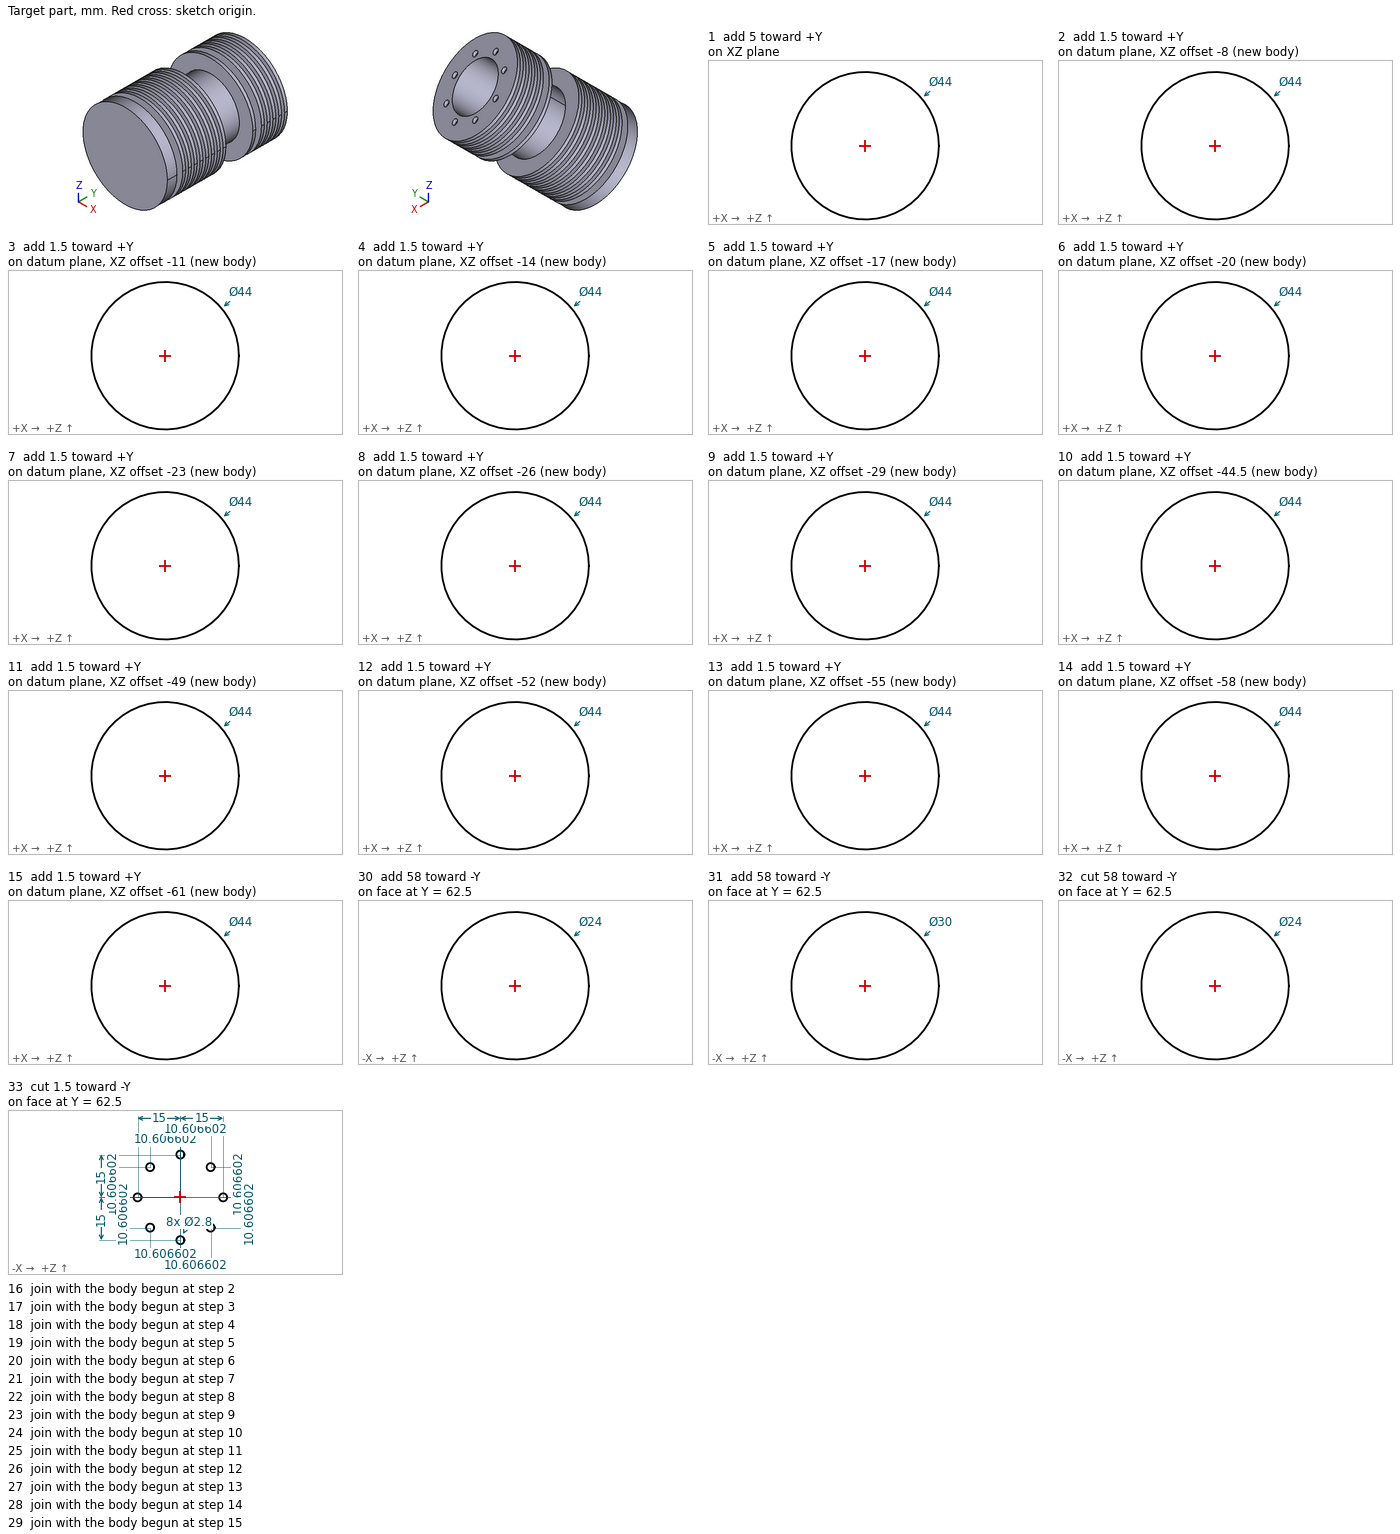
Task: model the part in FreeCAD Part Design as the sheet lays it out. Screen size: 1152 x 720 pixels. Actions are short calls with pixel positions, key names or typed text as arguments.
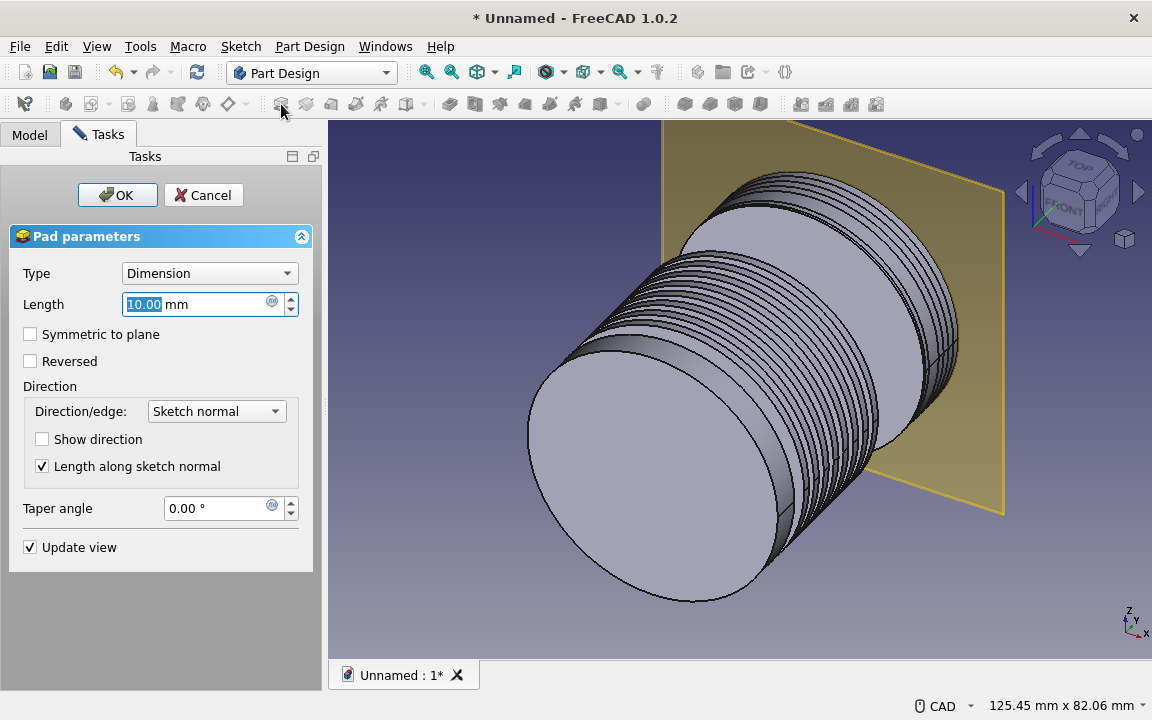
text(1.5)
key(Tab)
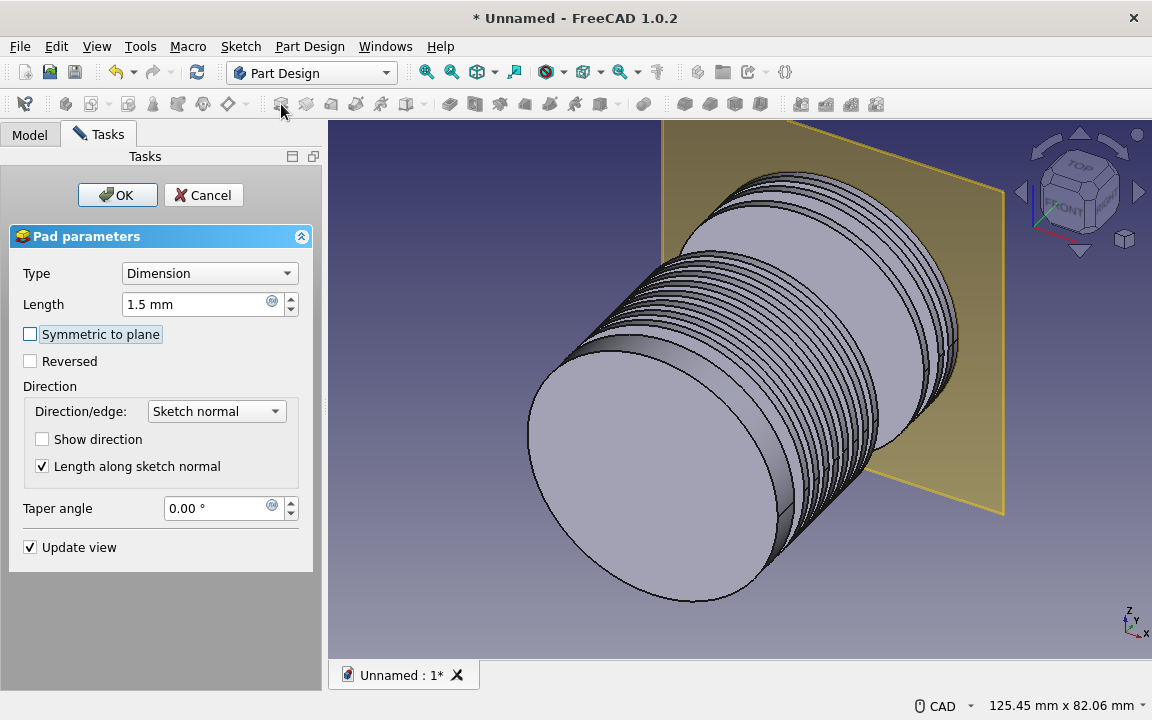
click(31, 361)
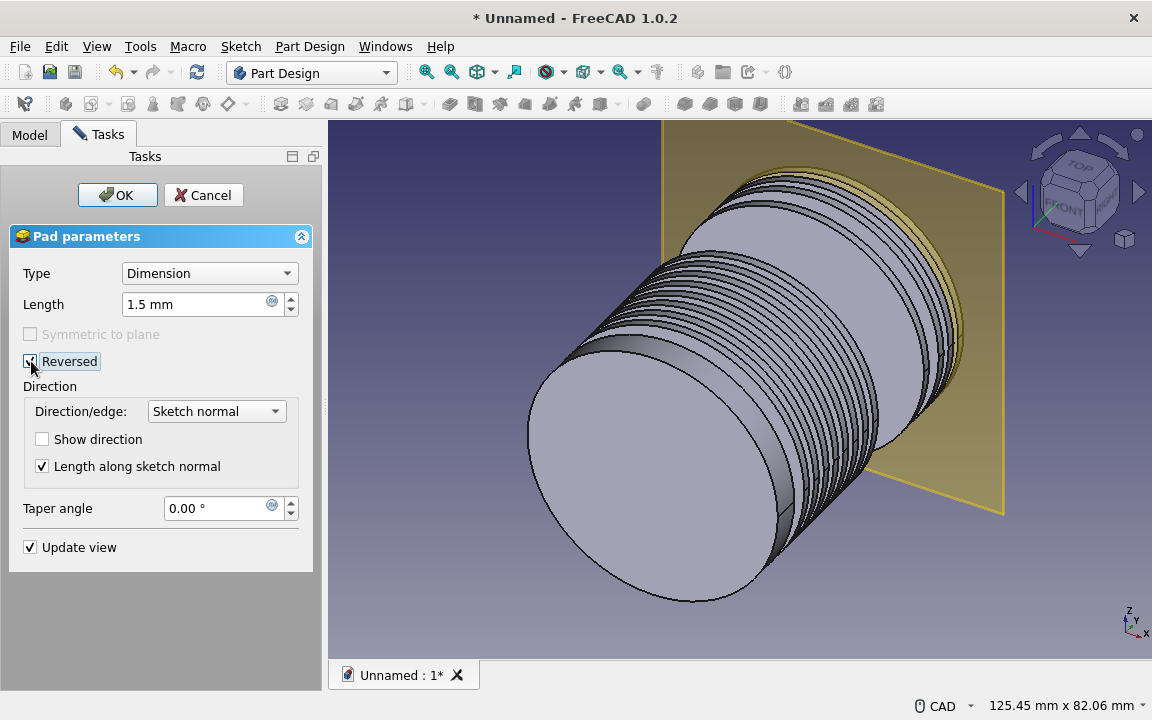
click(118, 195)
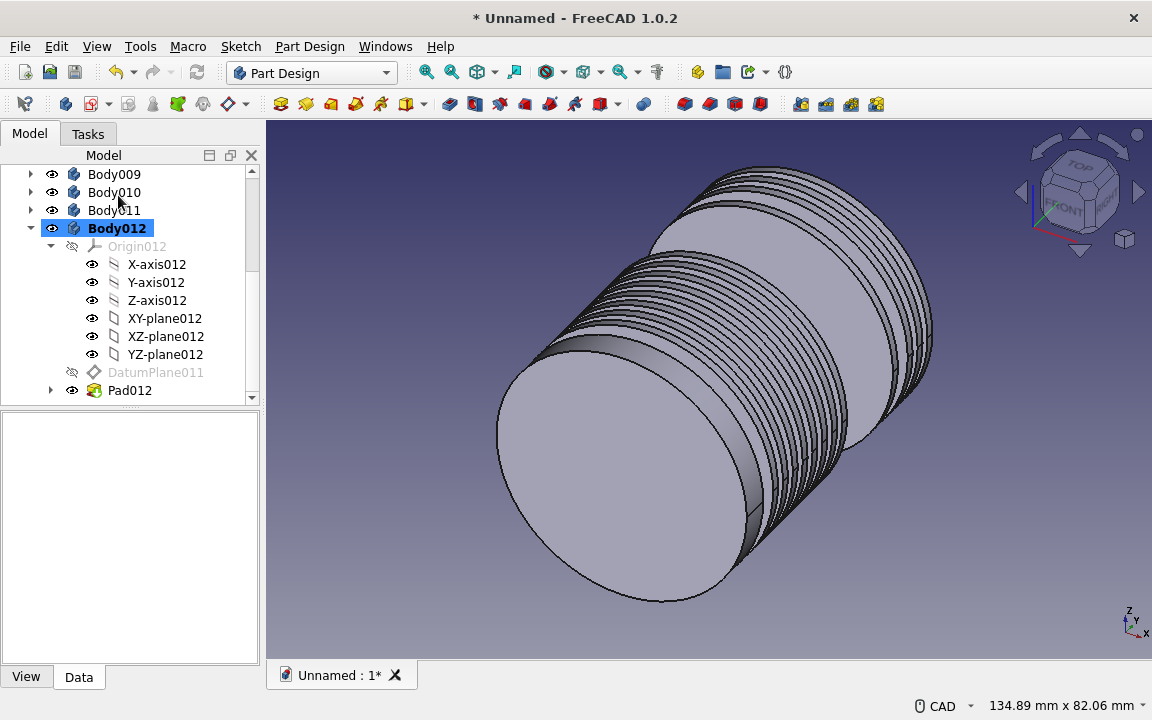
click(66, 104)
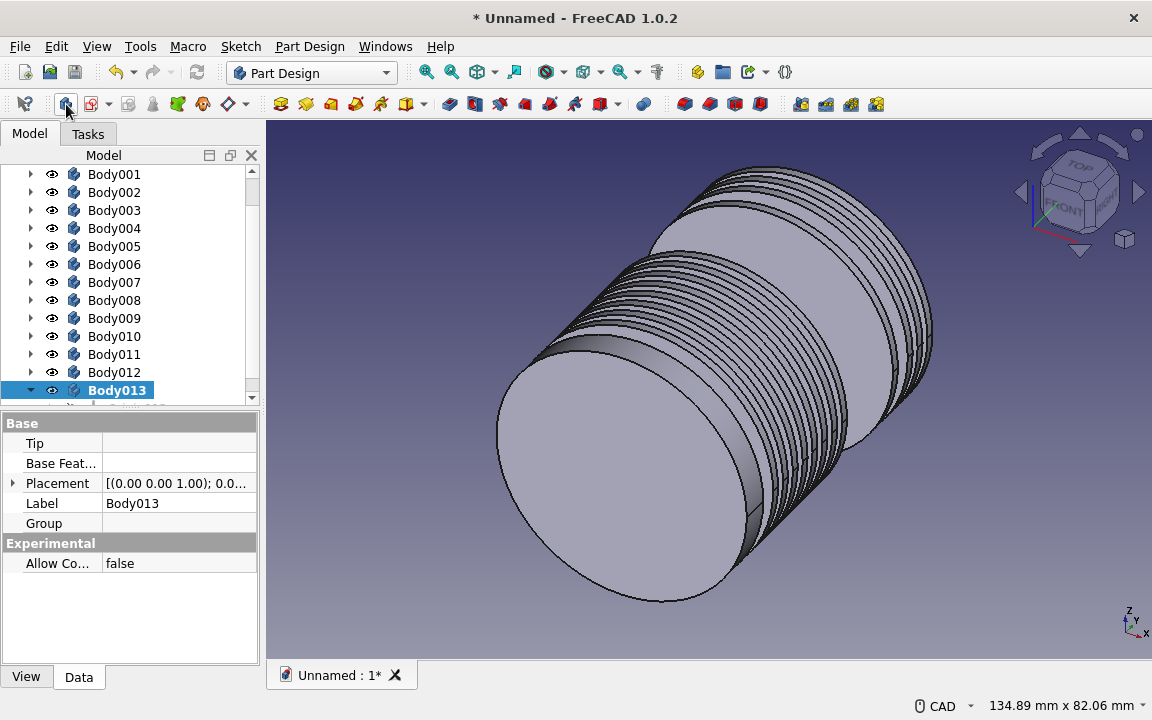
scroll(121, 278, down, 3)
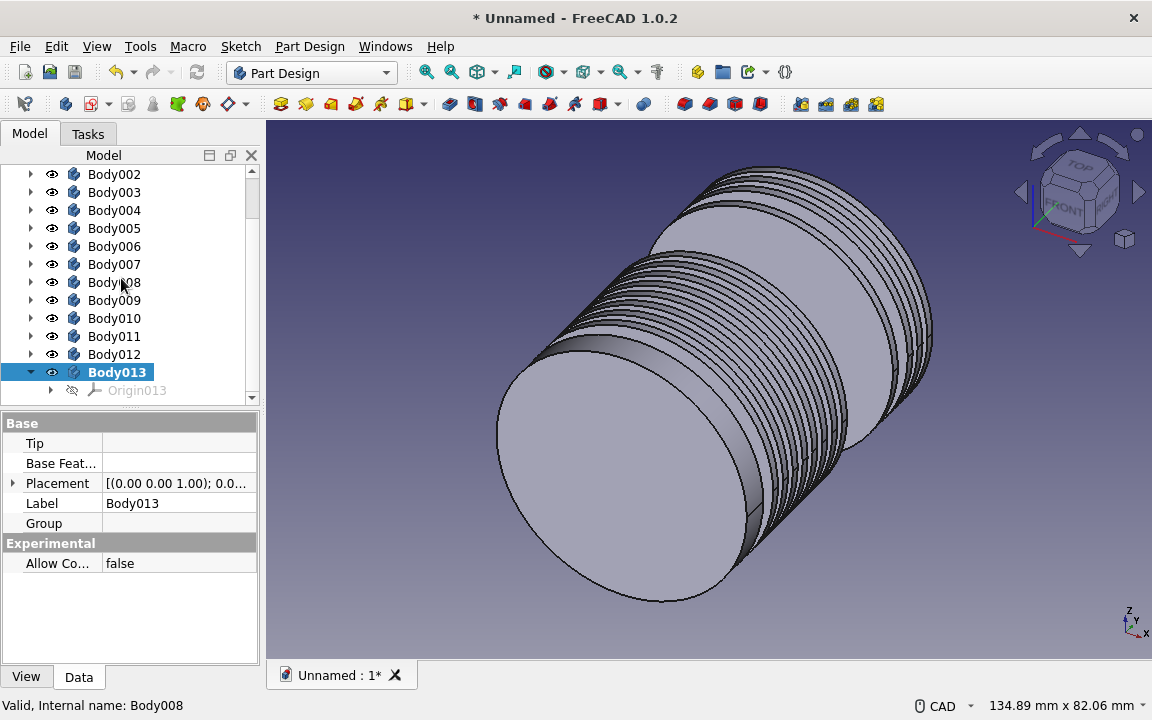
click(51, 390)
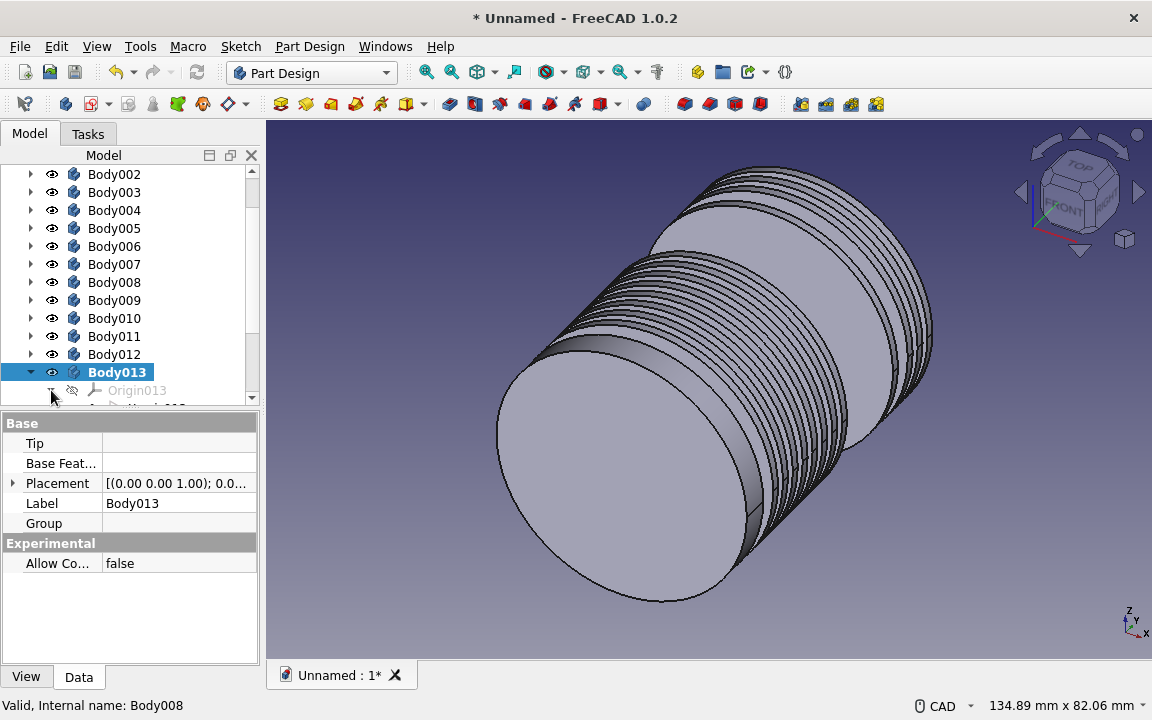
scroll(121, 278, down, 3)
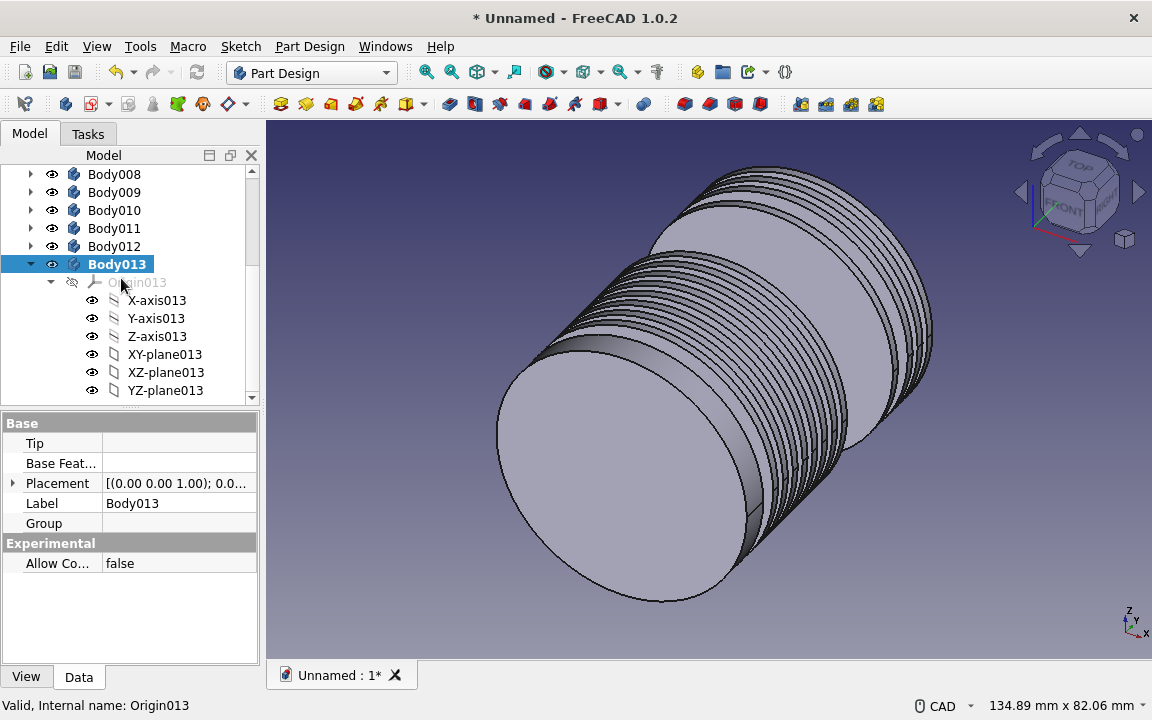
click(137, 372)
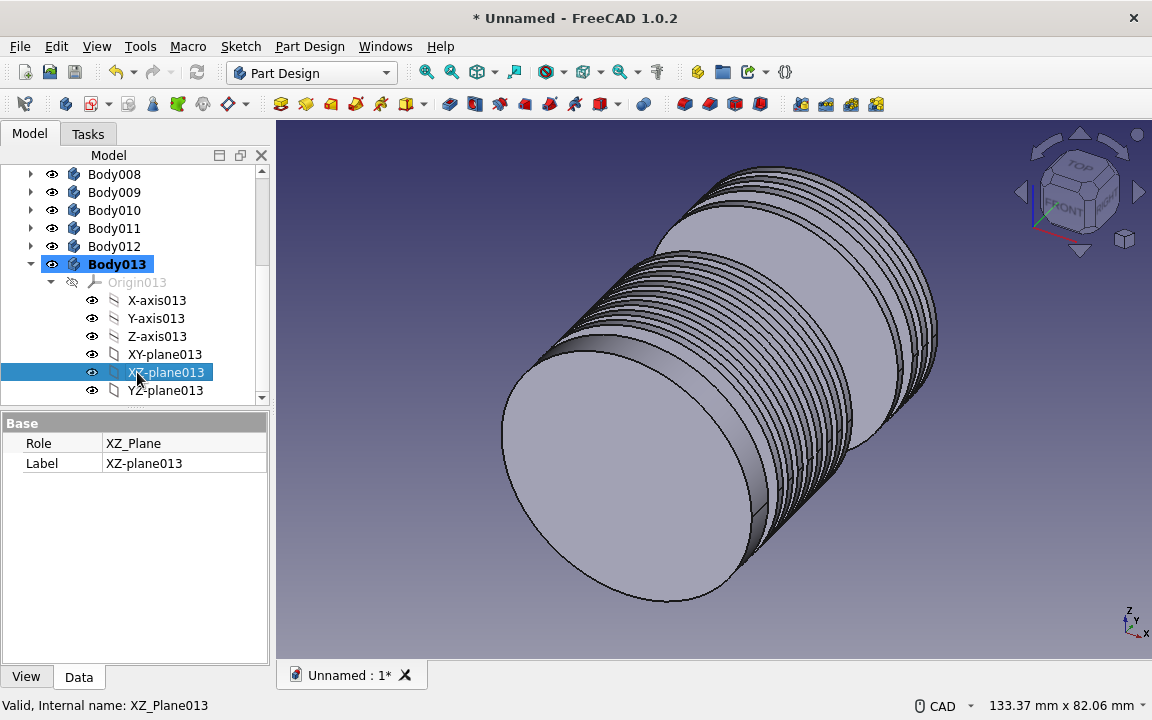
click(228, 104)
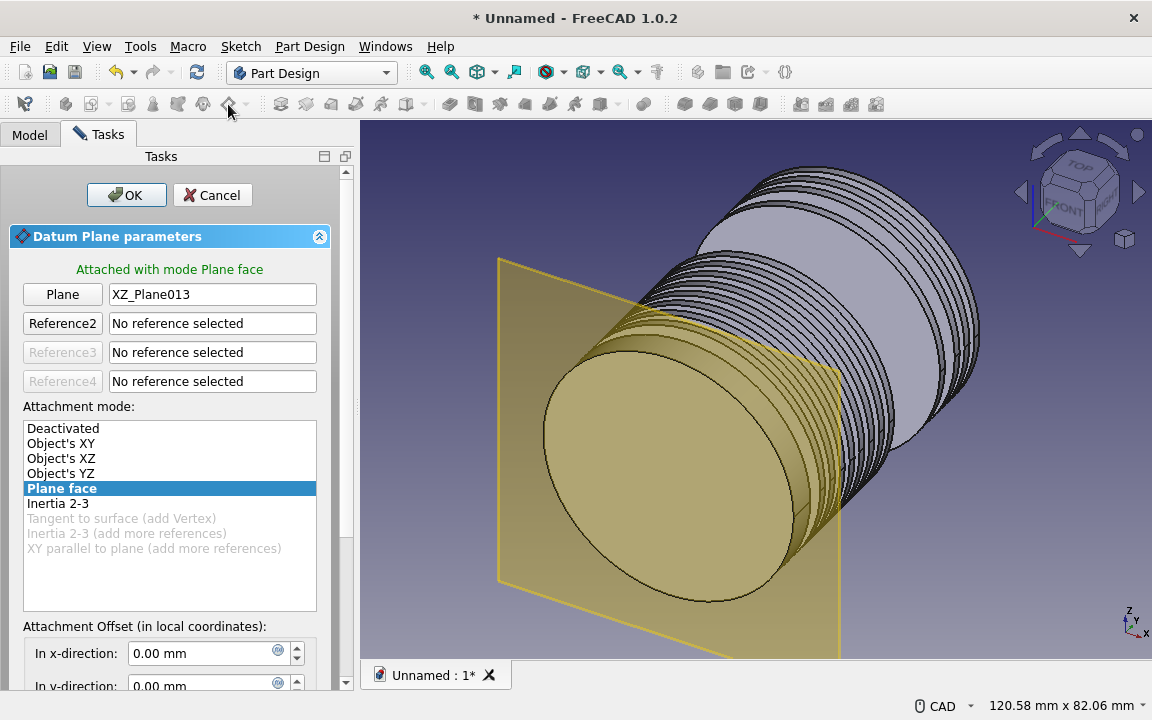
scroll(346, 428, down, 2)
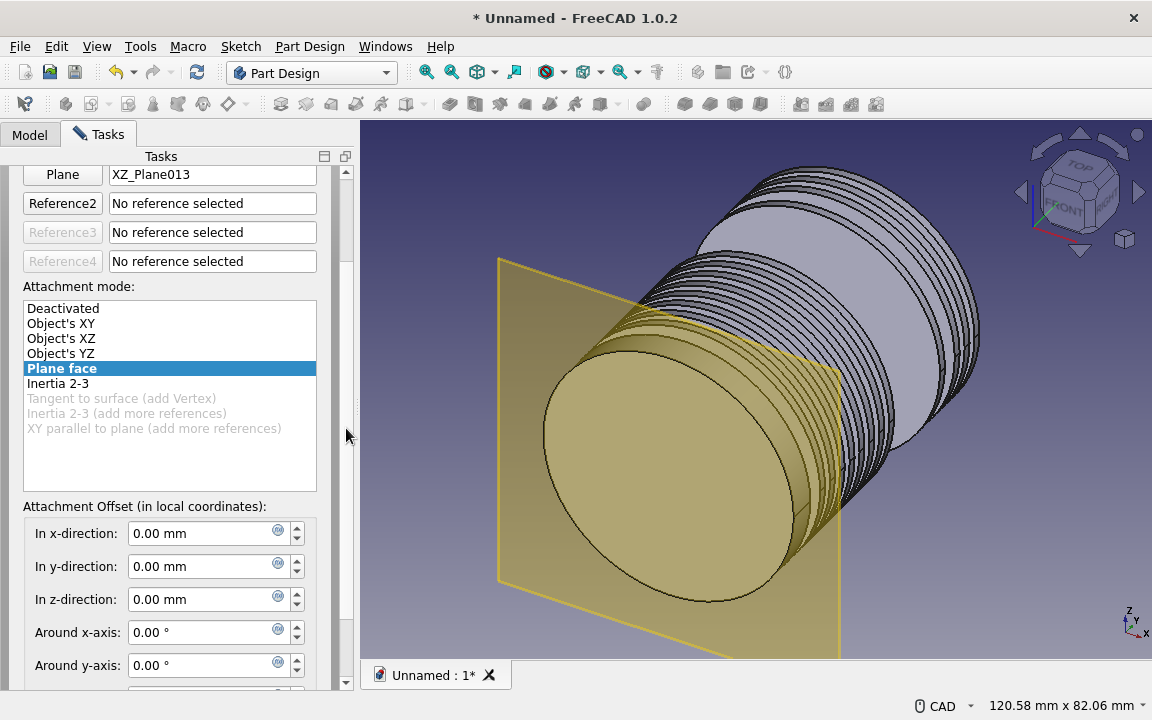
triple_click(210, 600)